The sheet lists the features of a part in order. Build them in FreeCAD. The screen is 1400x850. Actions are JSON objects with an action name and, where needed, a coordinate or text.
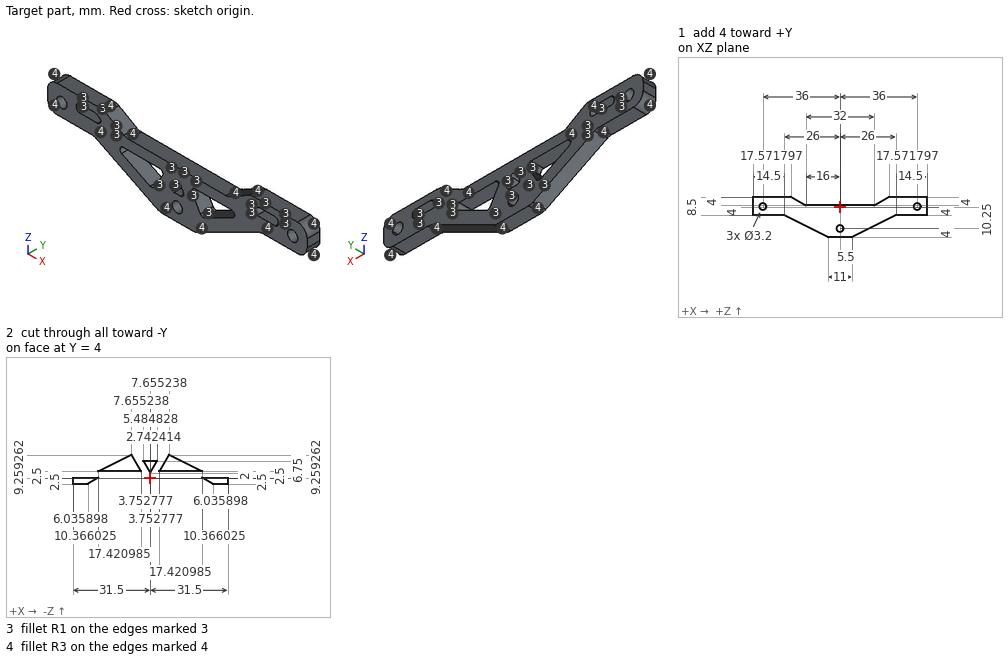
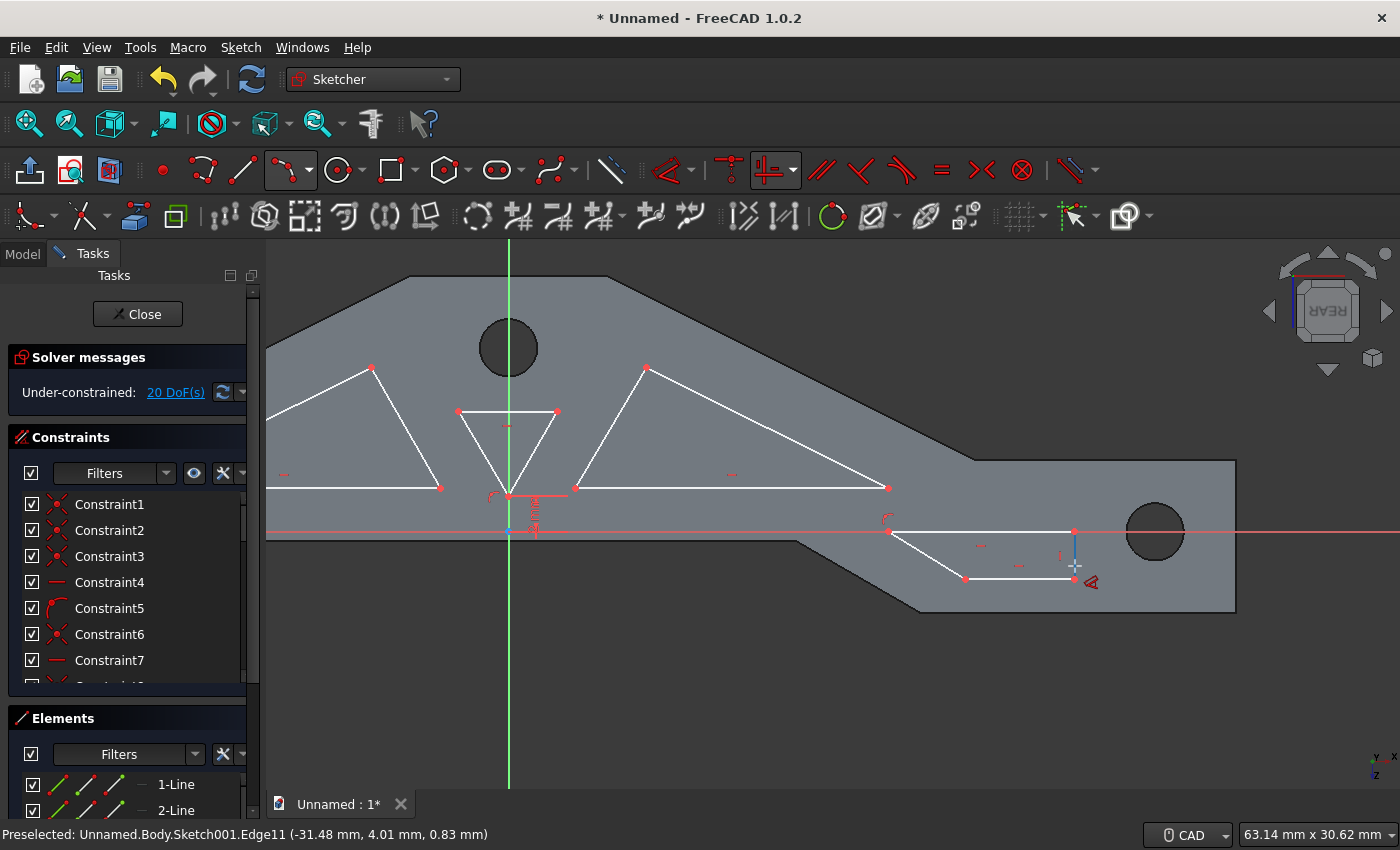
{"action": "left_click", "coordinate": [1075, 565]}
{"action": "left_click", "coordinate": [1109, 556]}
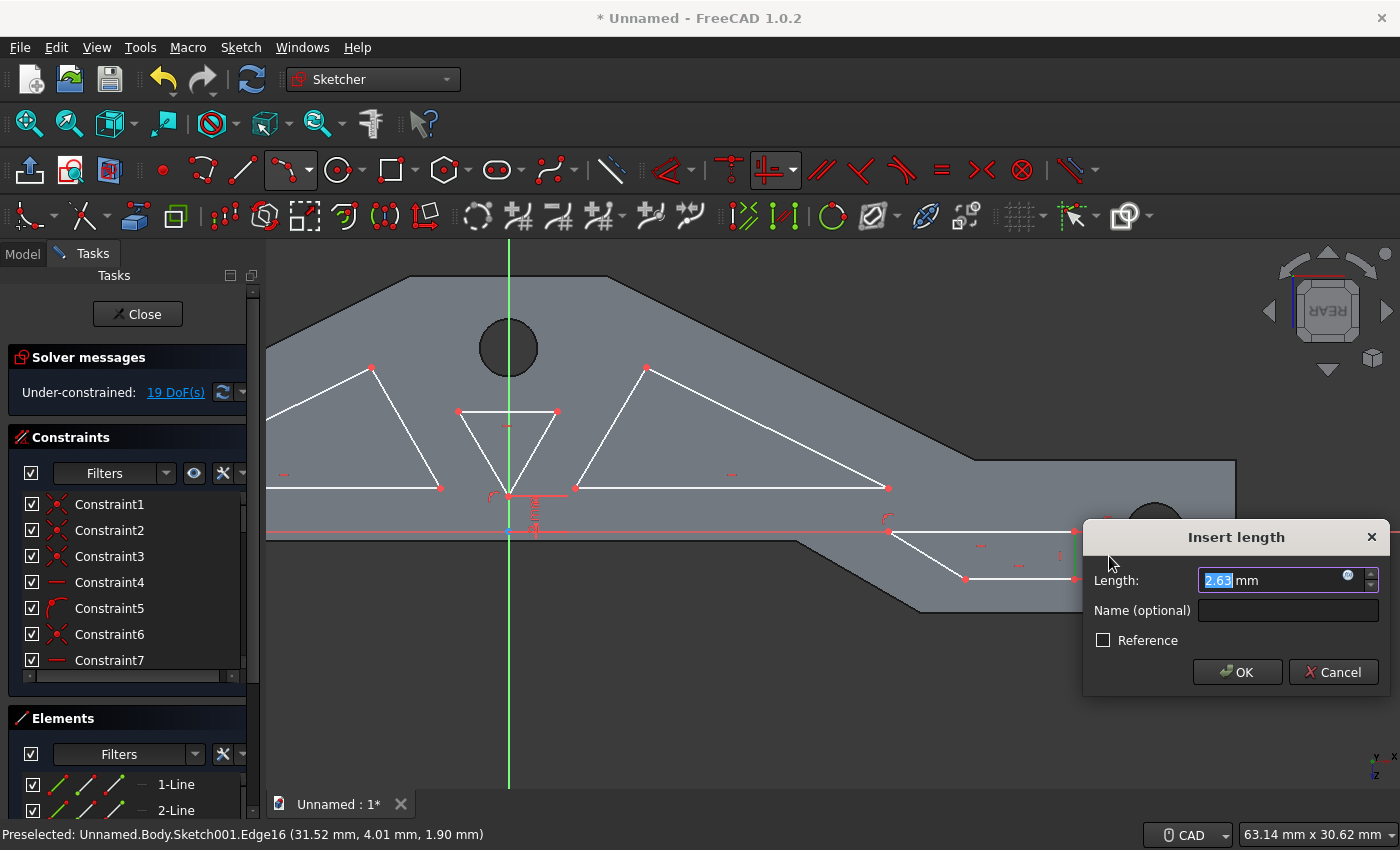
{"action": "type", "text": "2.5"}
{"action": "key", "text": "Return"}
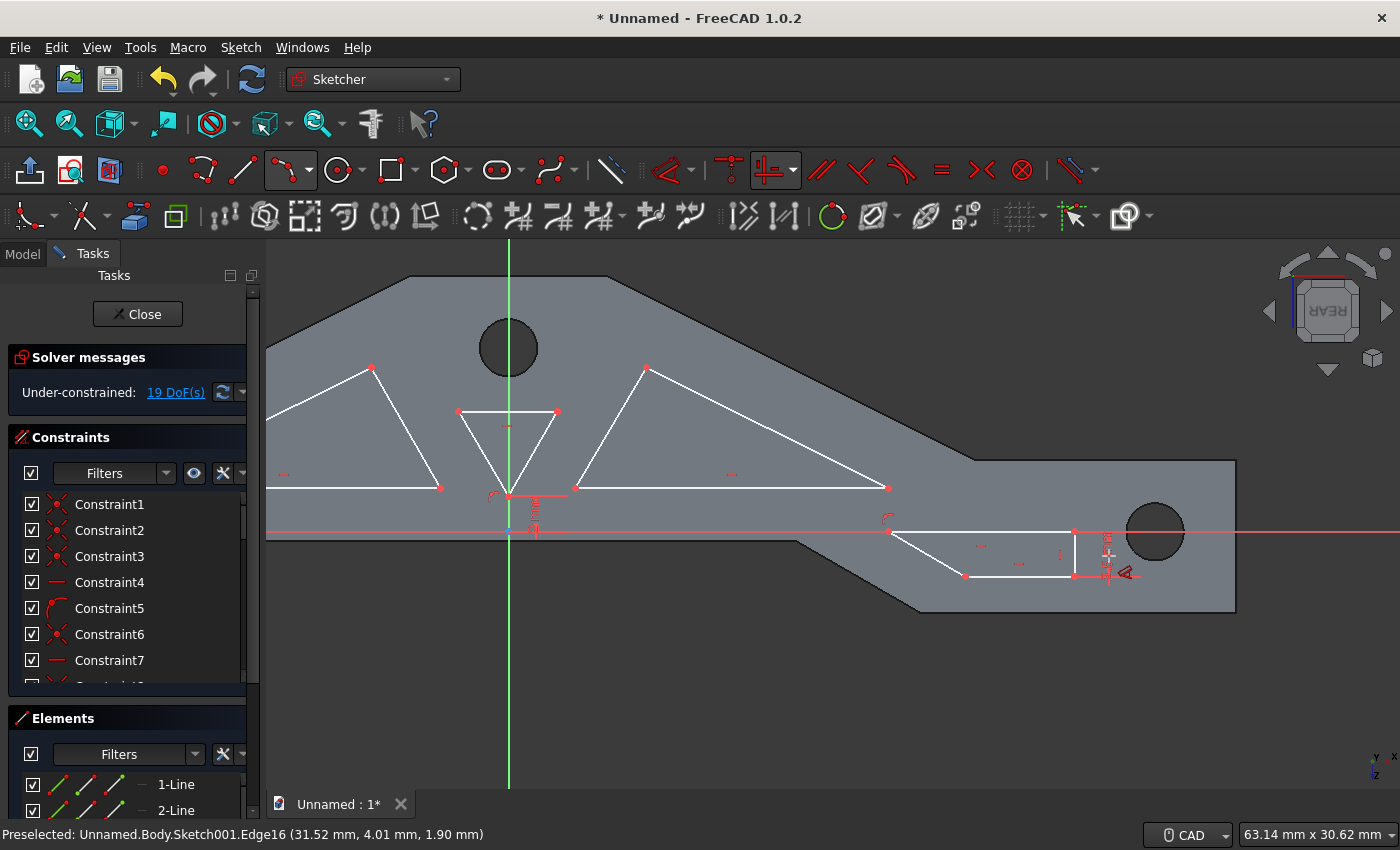
{"action": "left_click", "coordinate": [440, 488]}
{"action": "left_click", "coordinate": [406, 510]}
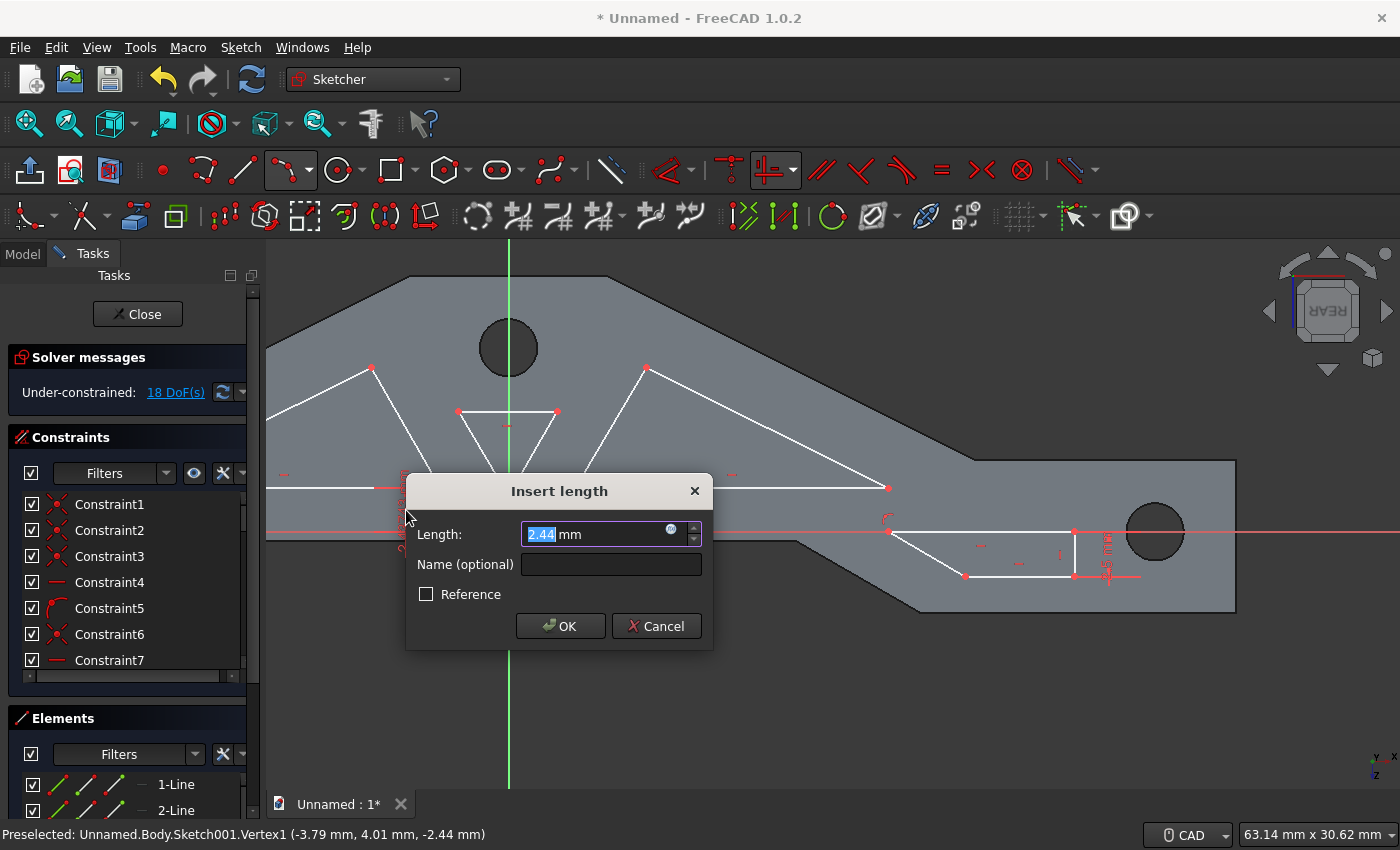
{"action": "type", "text": "2.5"}
{"action": "key", "text": "Return"}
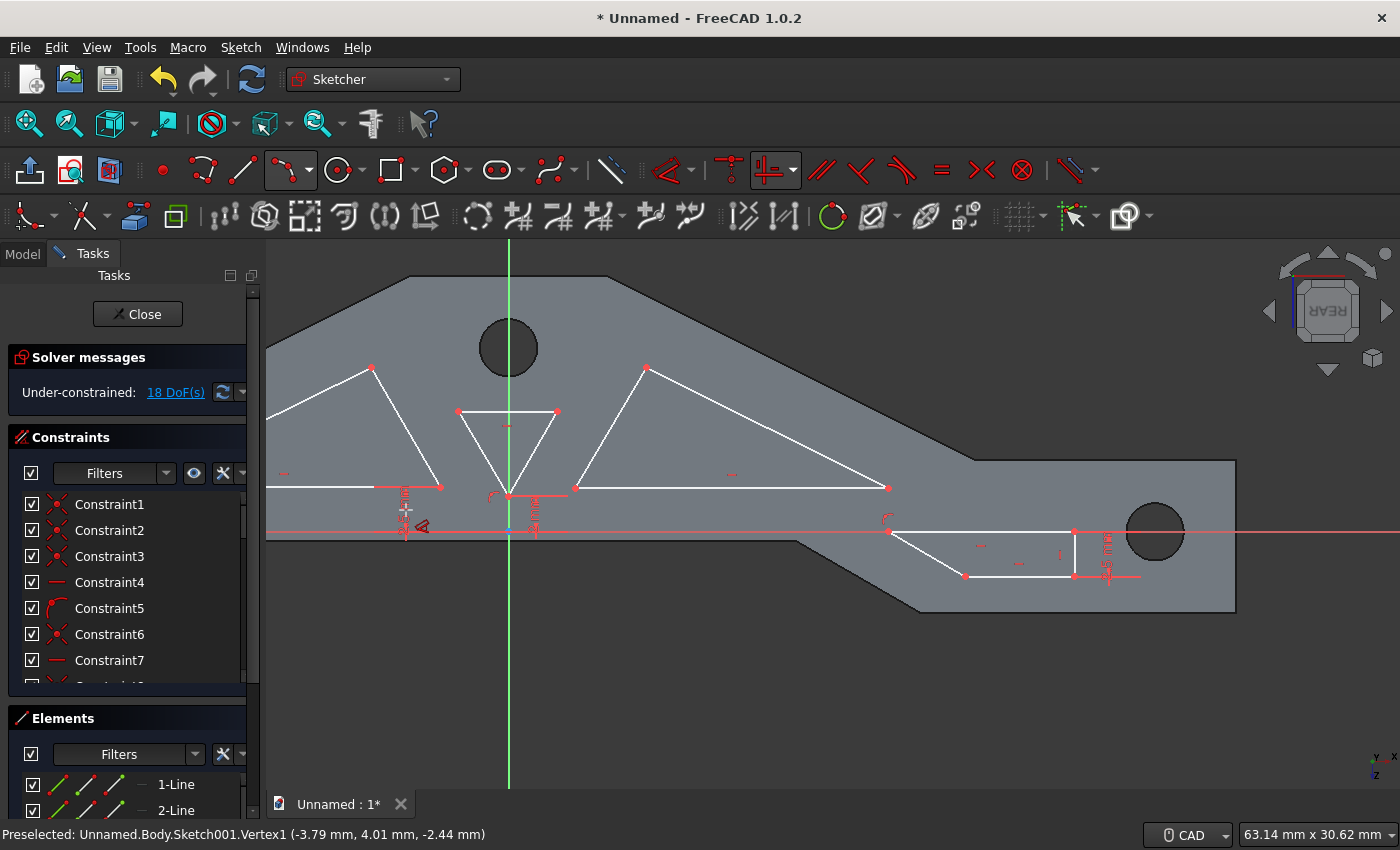
{"action": "left_click", "coordinate": [575, 488]}
{"action": "left_click", "coordinate": [609, 510]}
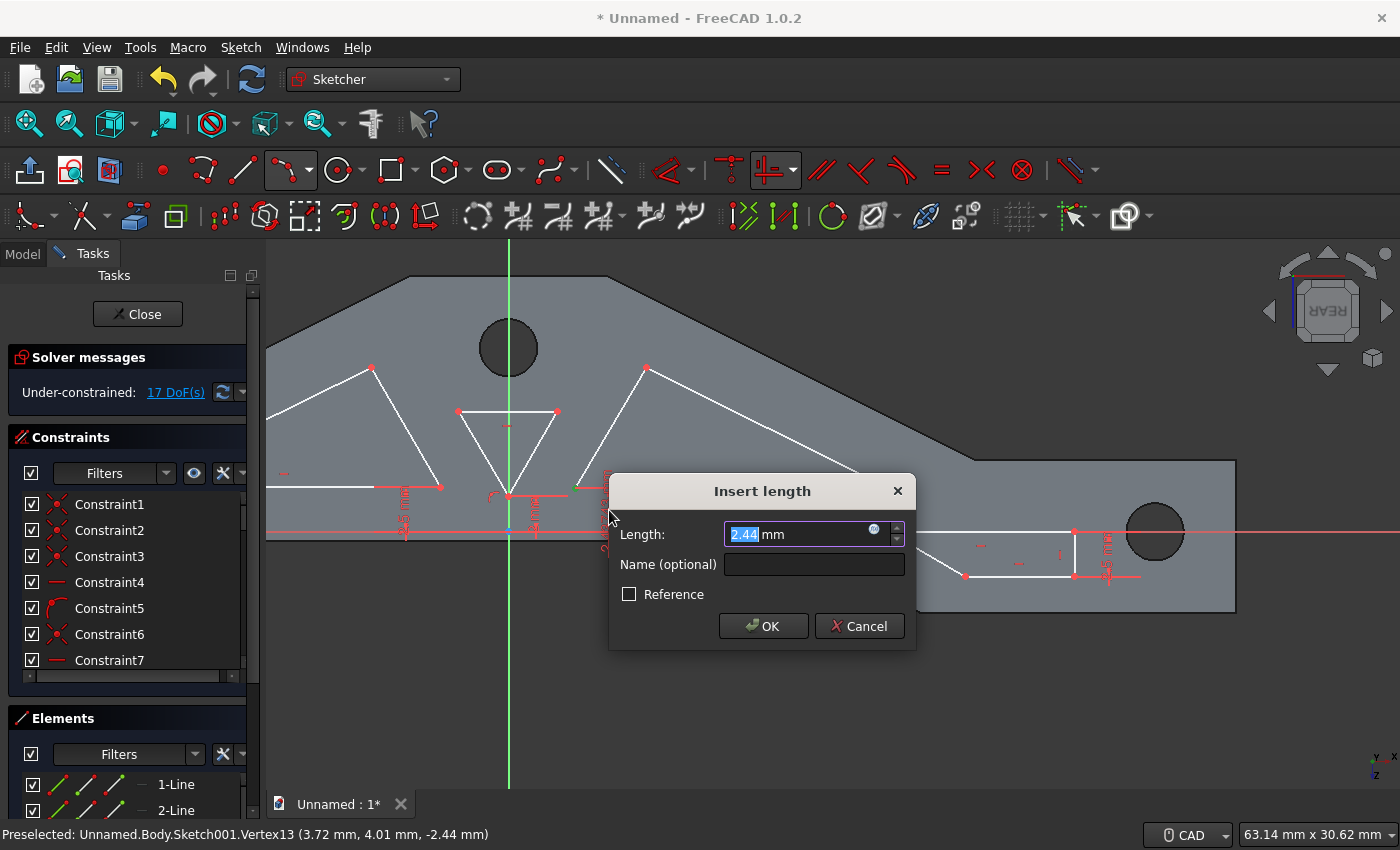
{"action": "type", "text": "2.5"}
{"action": "key", "text": "Return"}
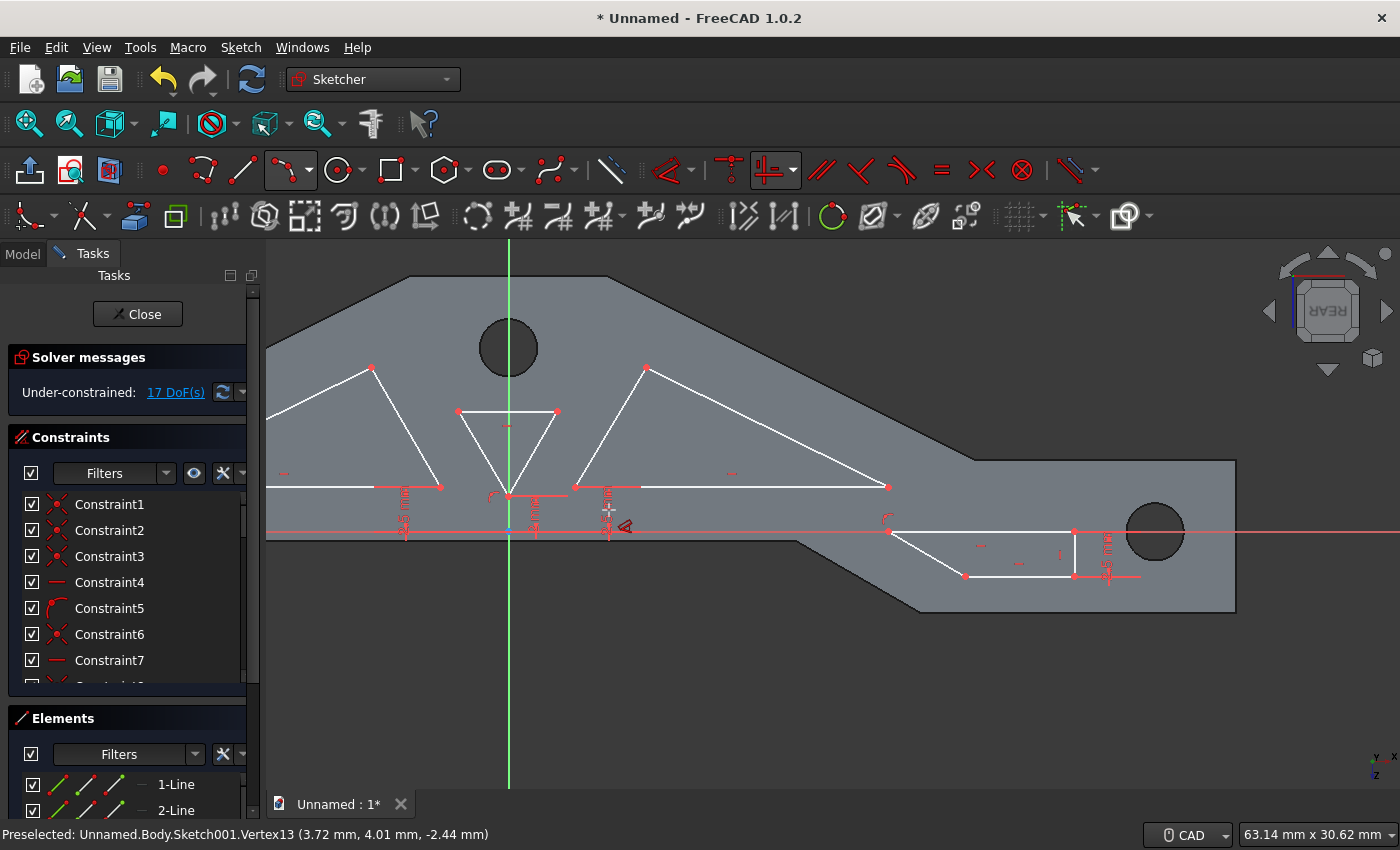
{"action": "left_click", "coordinate": [557, 412]}
{"action": "left_click", "coordinate": [591, 430]}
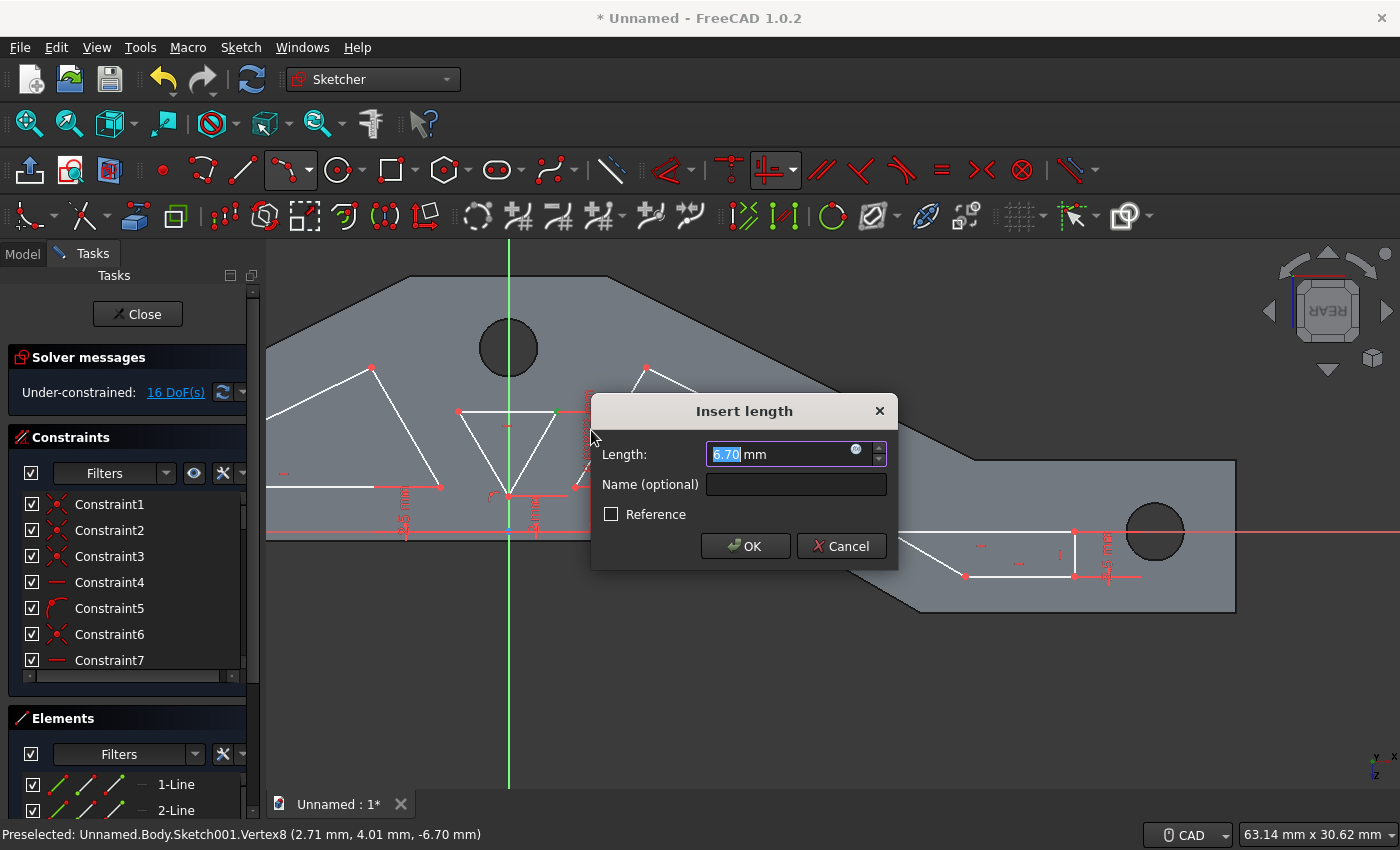
{"action": "type", "text": "6.75"}
{"action": "key", "text": "Return"}